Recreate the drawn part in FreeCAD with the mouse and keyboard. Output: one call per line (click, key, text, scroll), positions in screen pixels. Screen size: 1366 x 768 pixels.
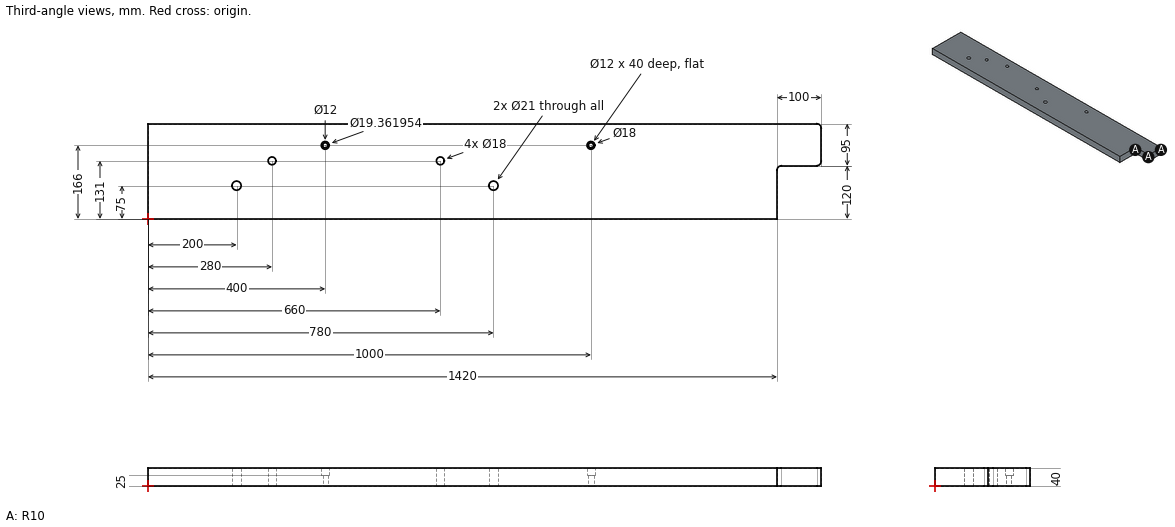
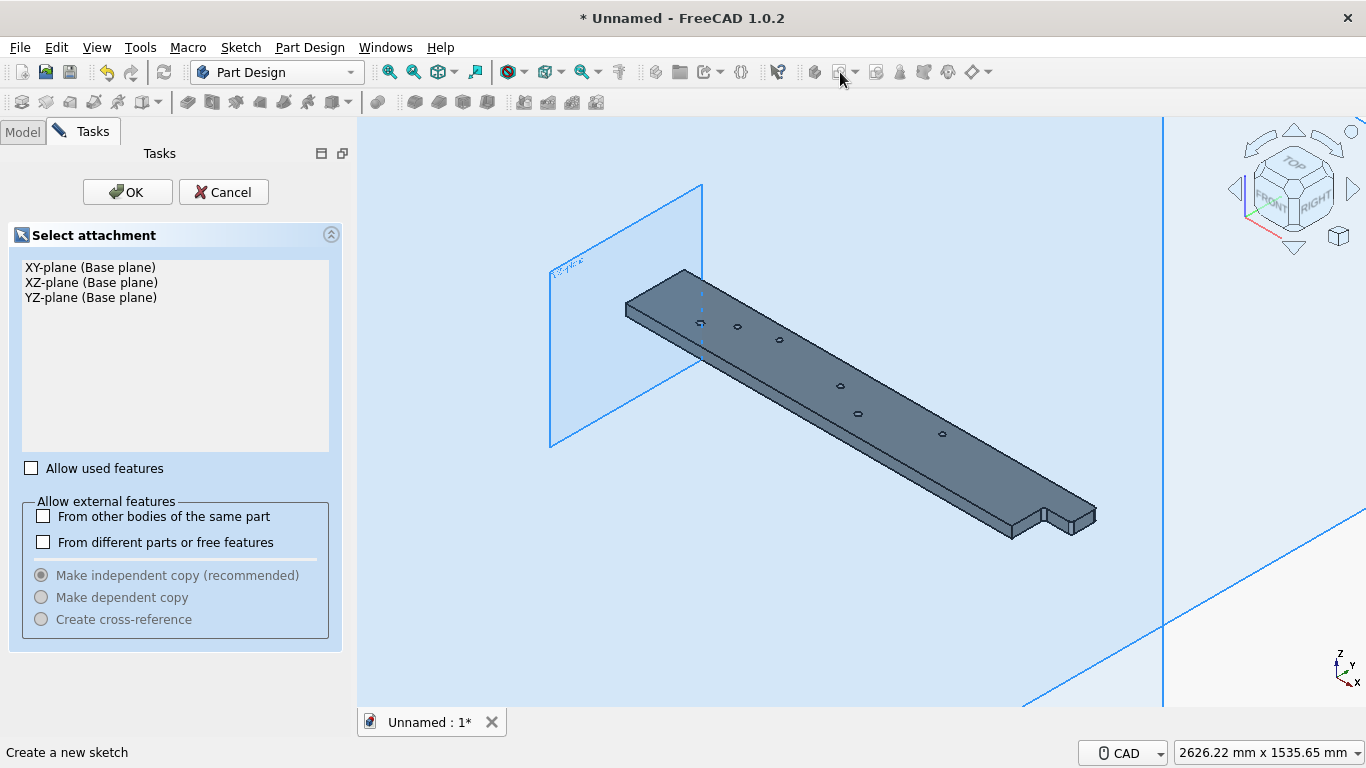
click(82, 268)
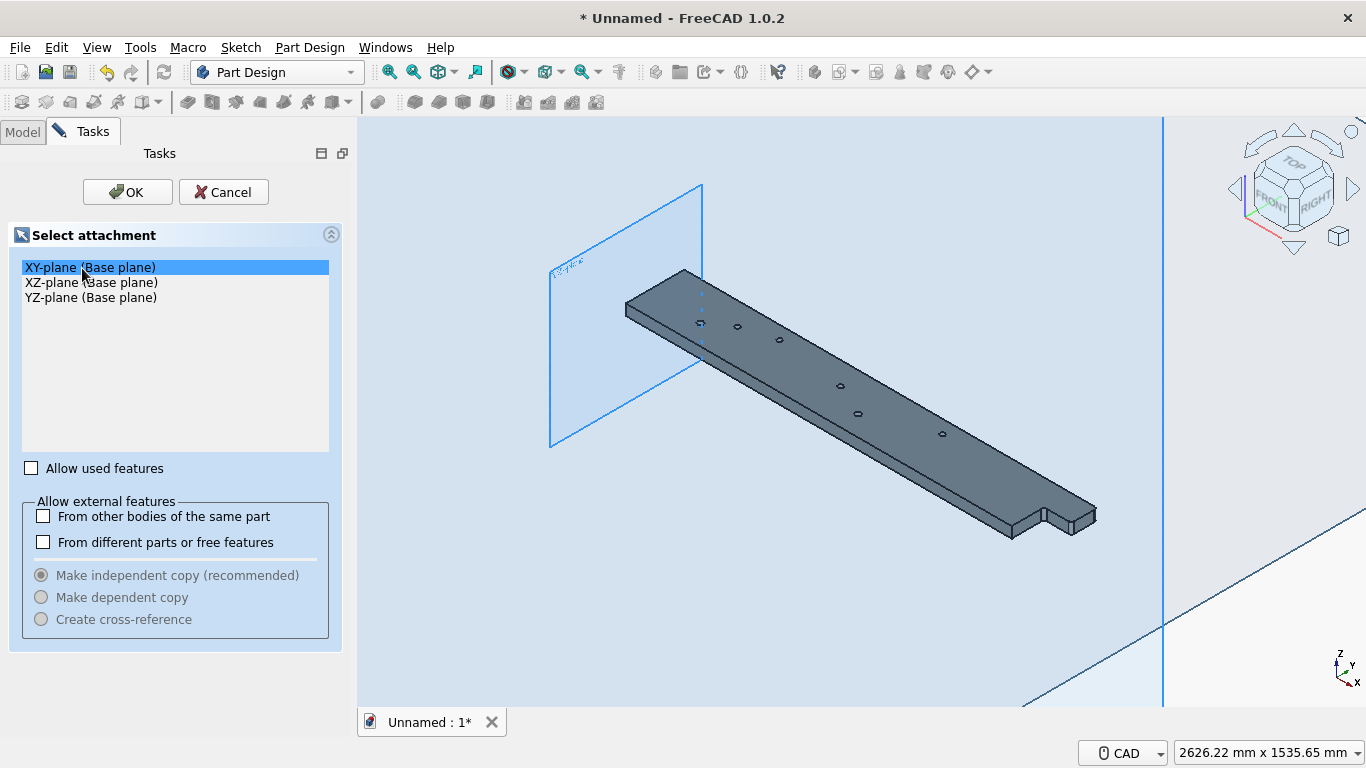
click(128, 192)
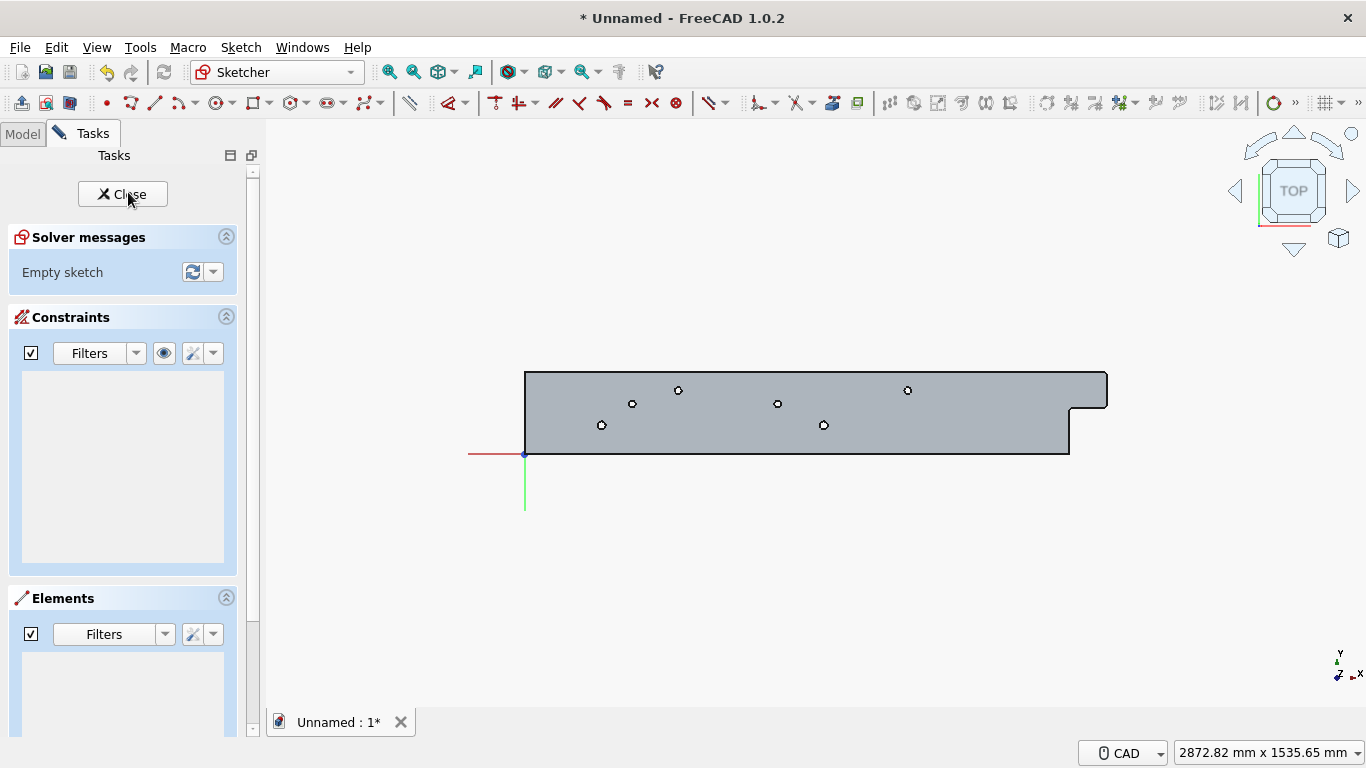
key(q)
key(s)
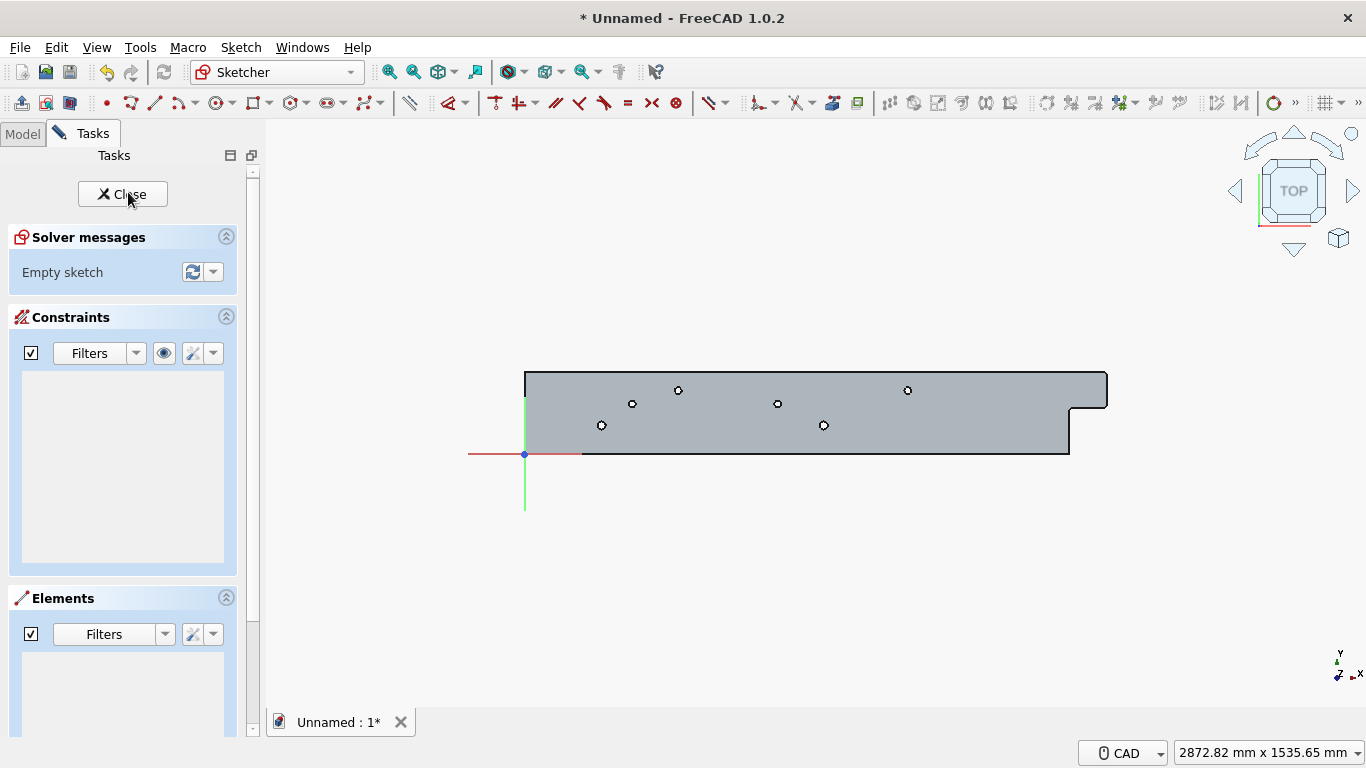
scroll(682, 430, up, 3)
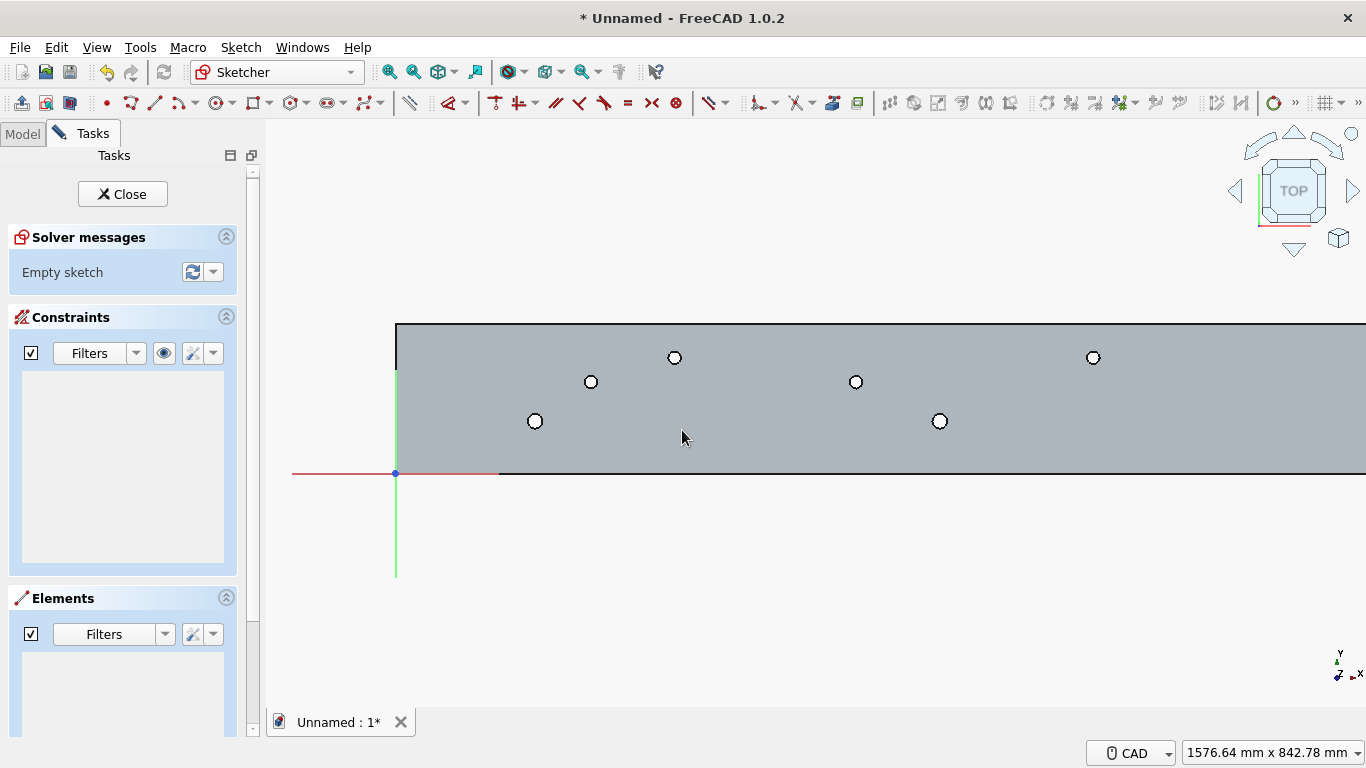
key(g)
key(c)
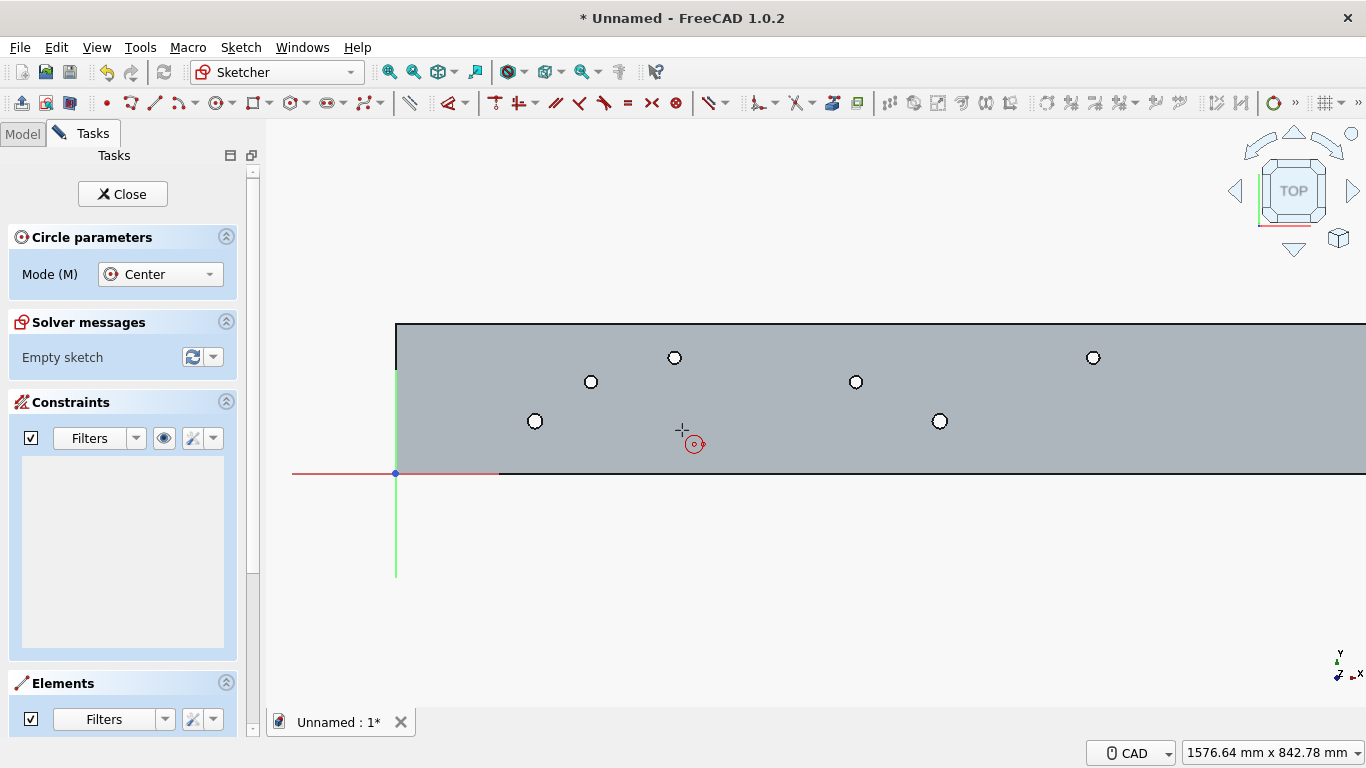
scroll(1093, 358, up, 7)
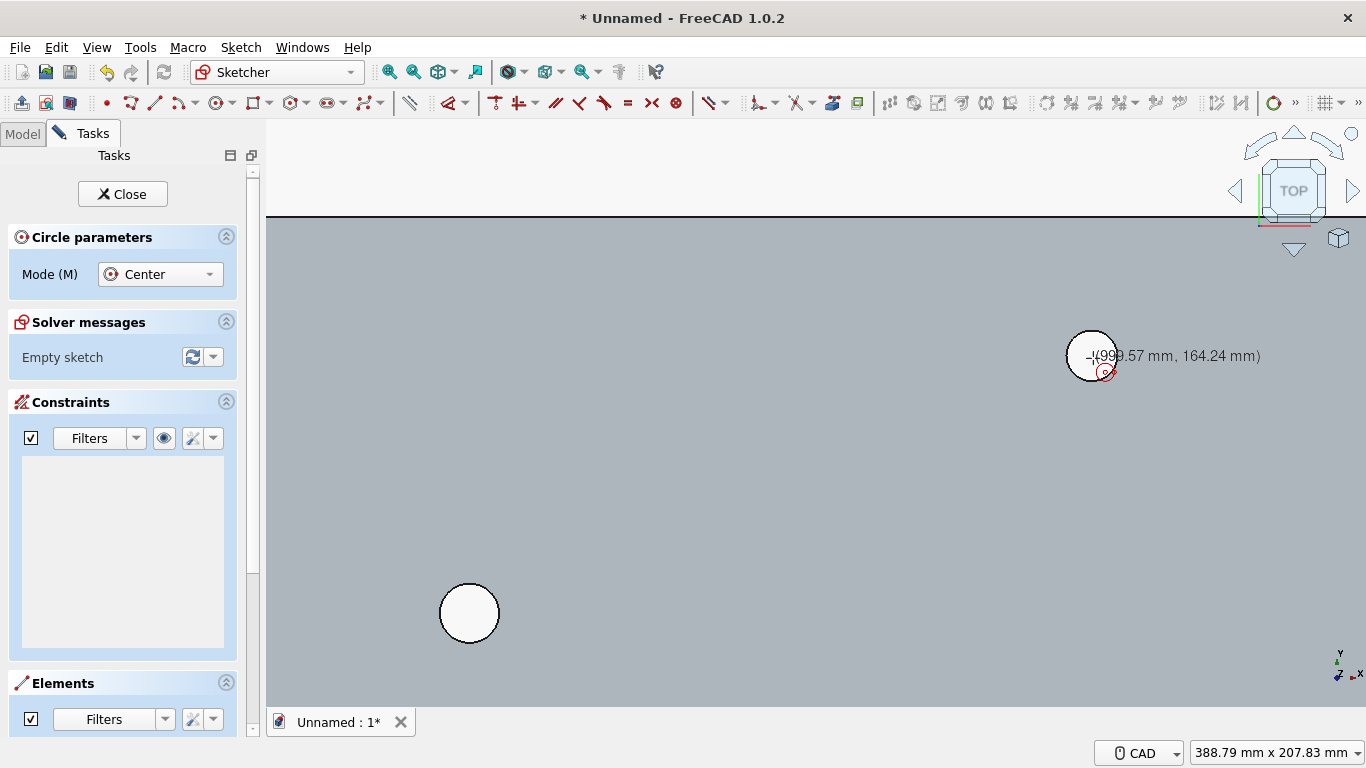
scroll(1094, 359, down, 7)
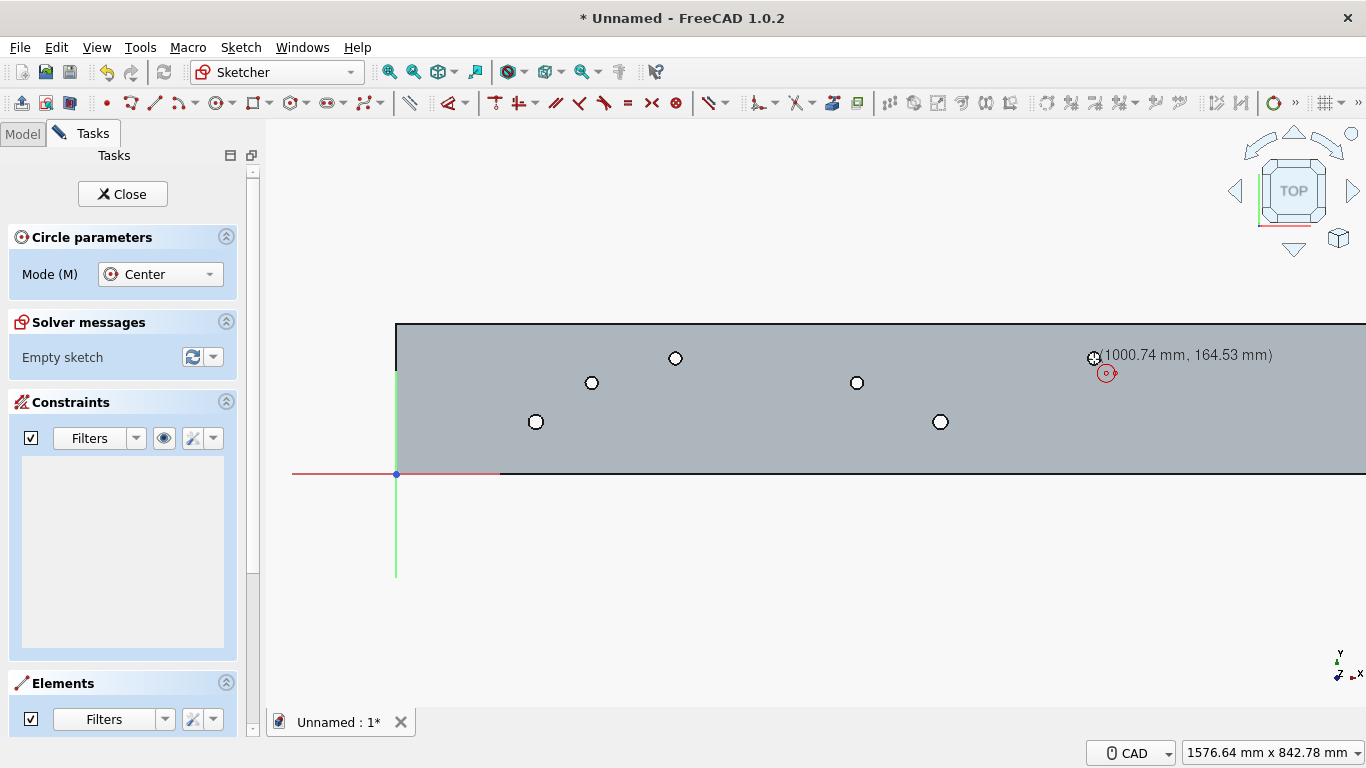
click(1094, 359)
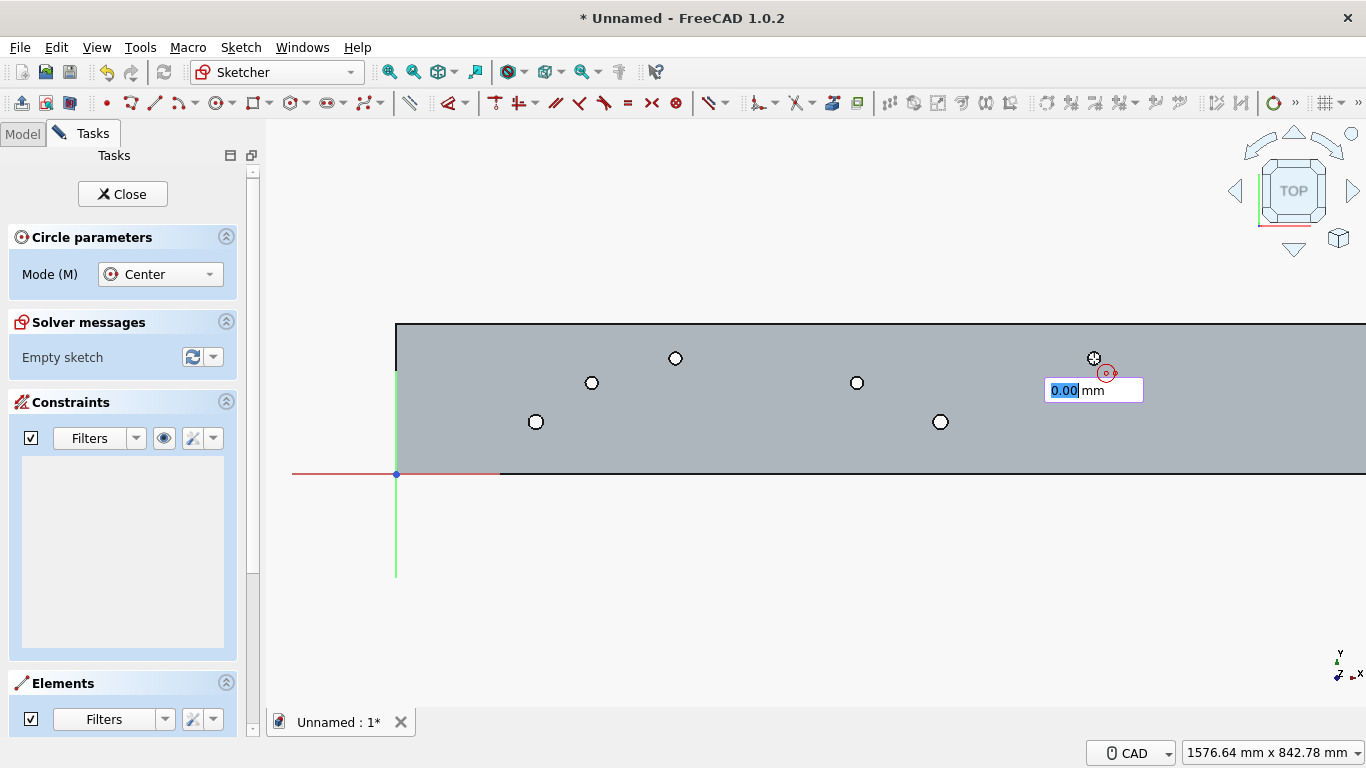
scroll(1098, 354, up, 5)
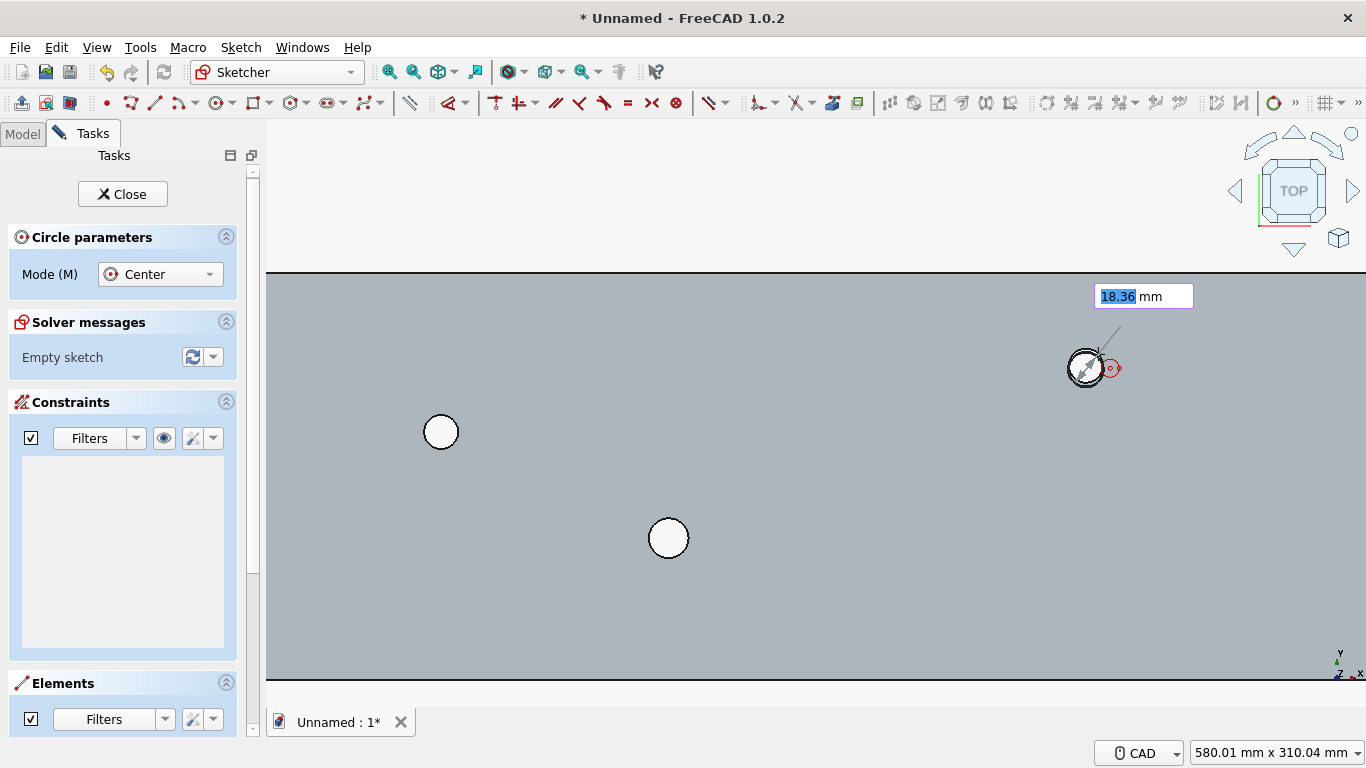
click(1098, 354)